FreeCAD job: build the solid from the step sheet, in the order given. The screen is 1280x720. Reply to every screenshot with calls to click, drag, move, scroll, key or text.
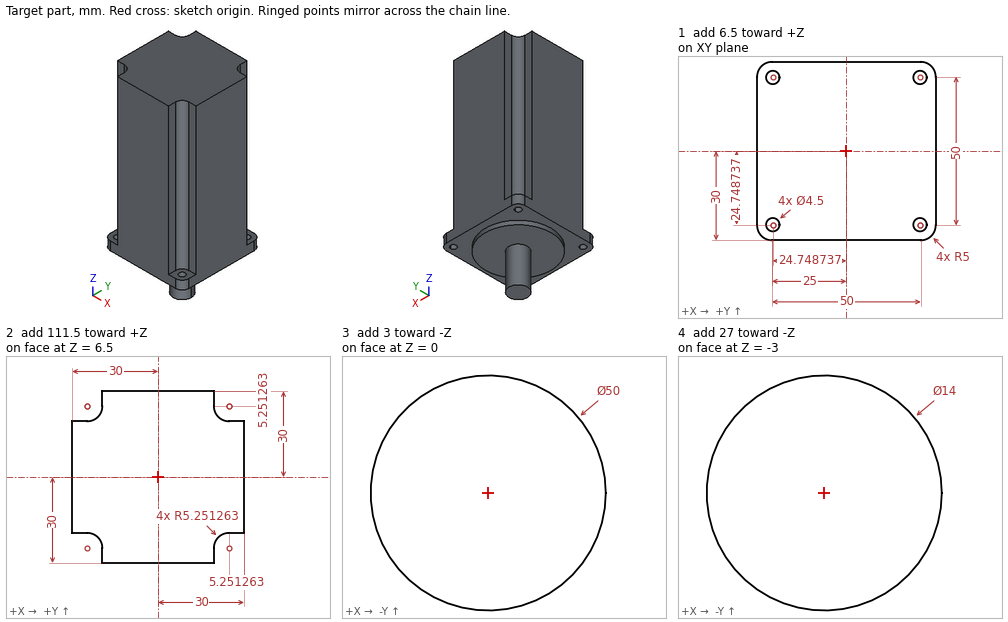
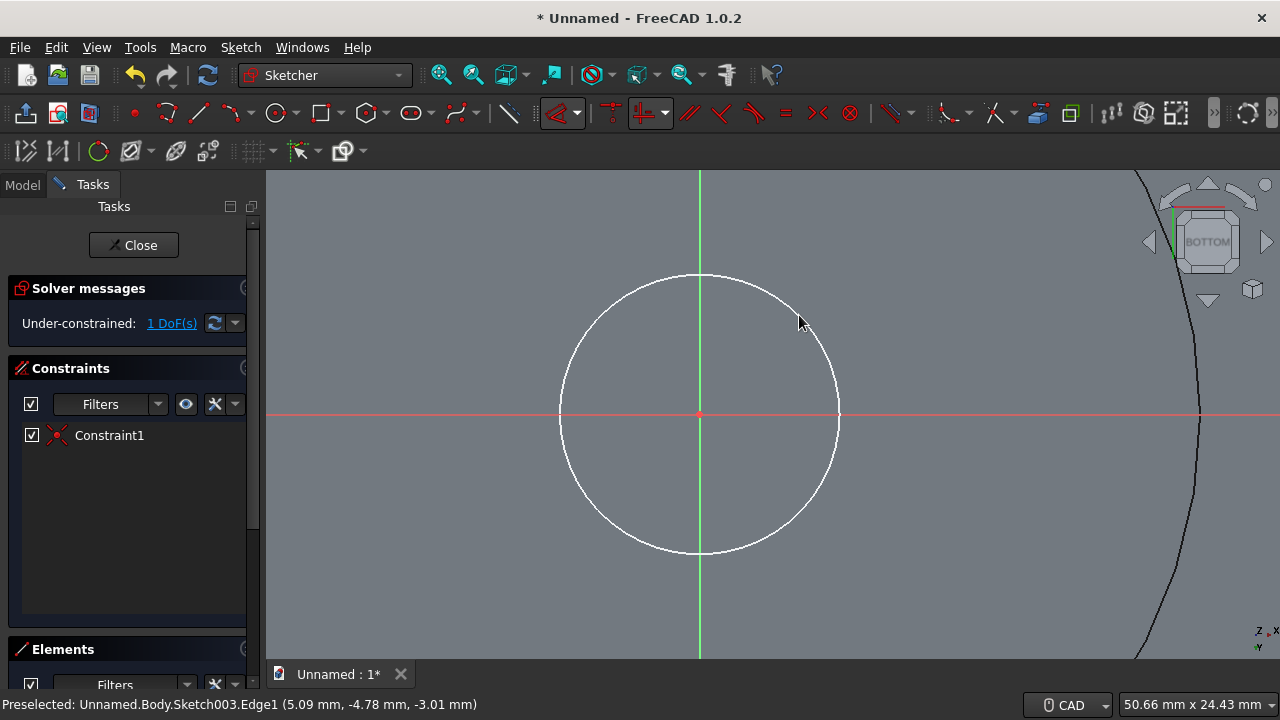
click(798, 315)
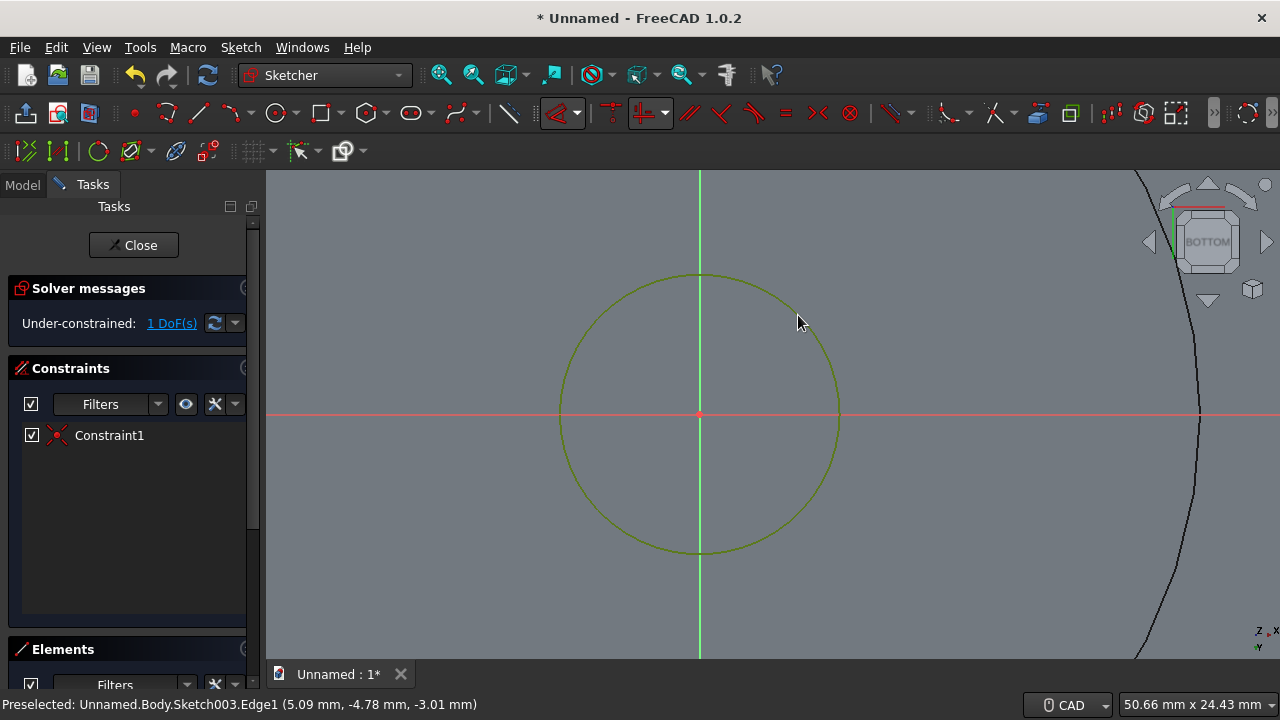
key(k)
key(o)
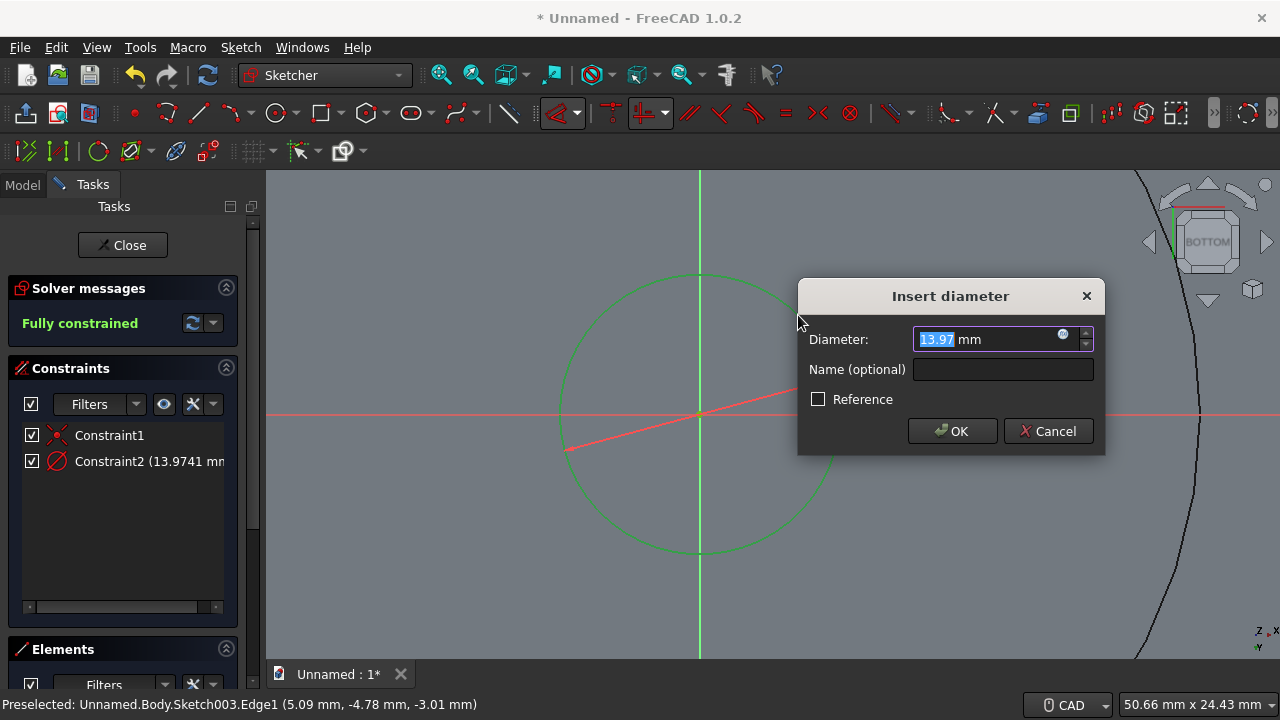
text(14)
key(Return)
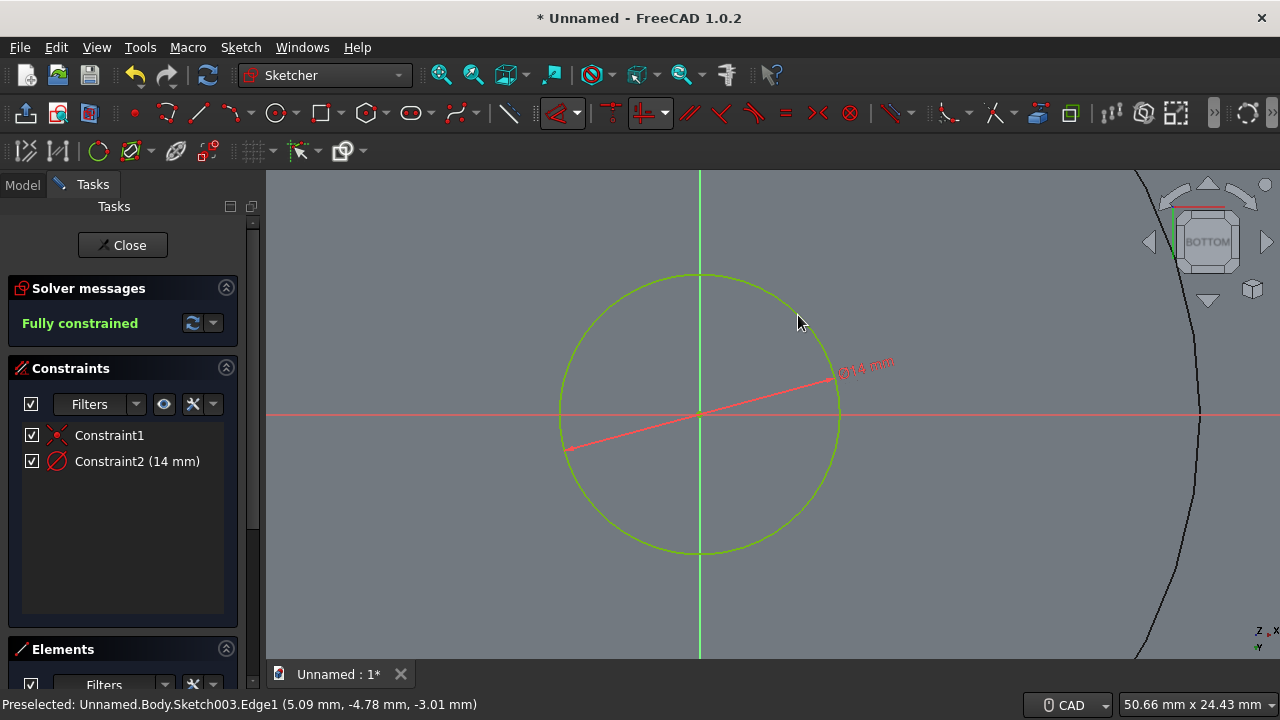
click(123, 245)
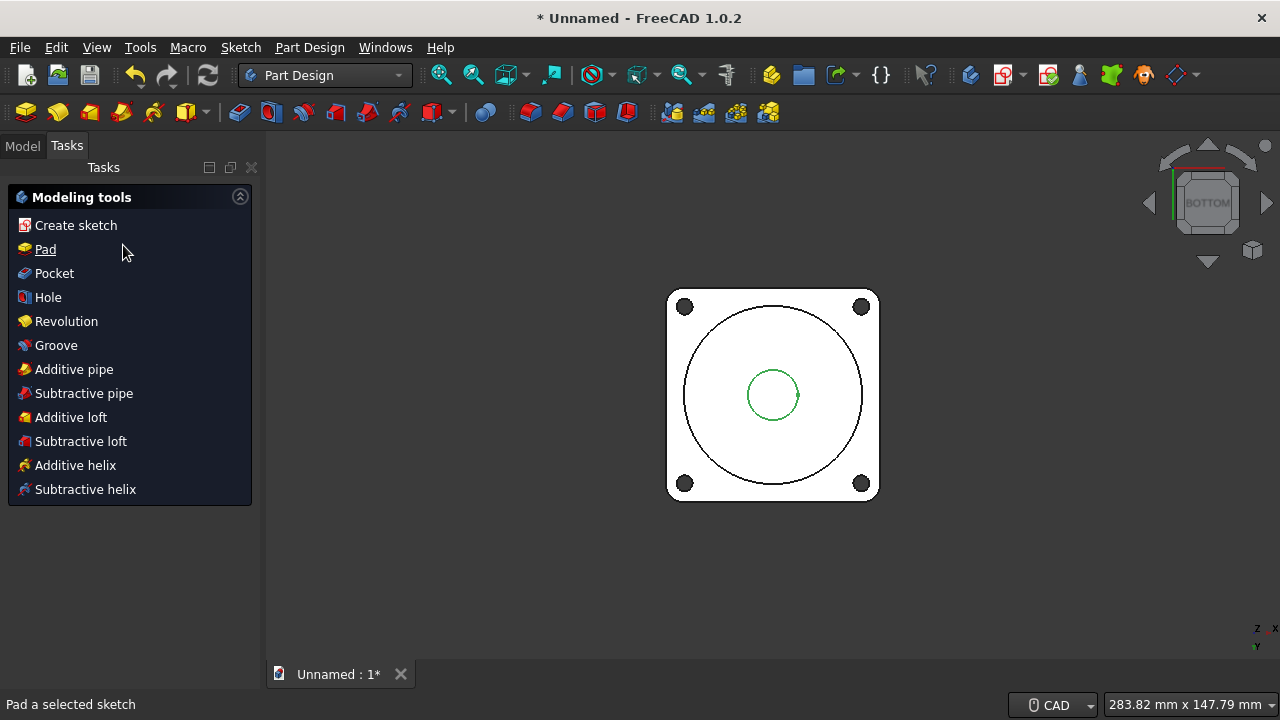
click(26, 112)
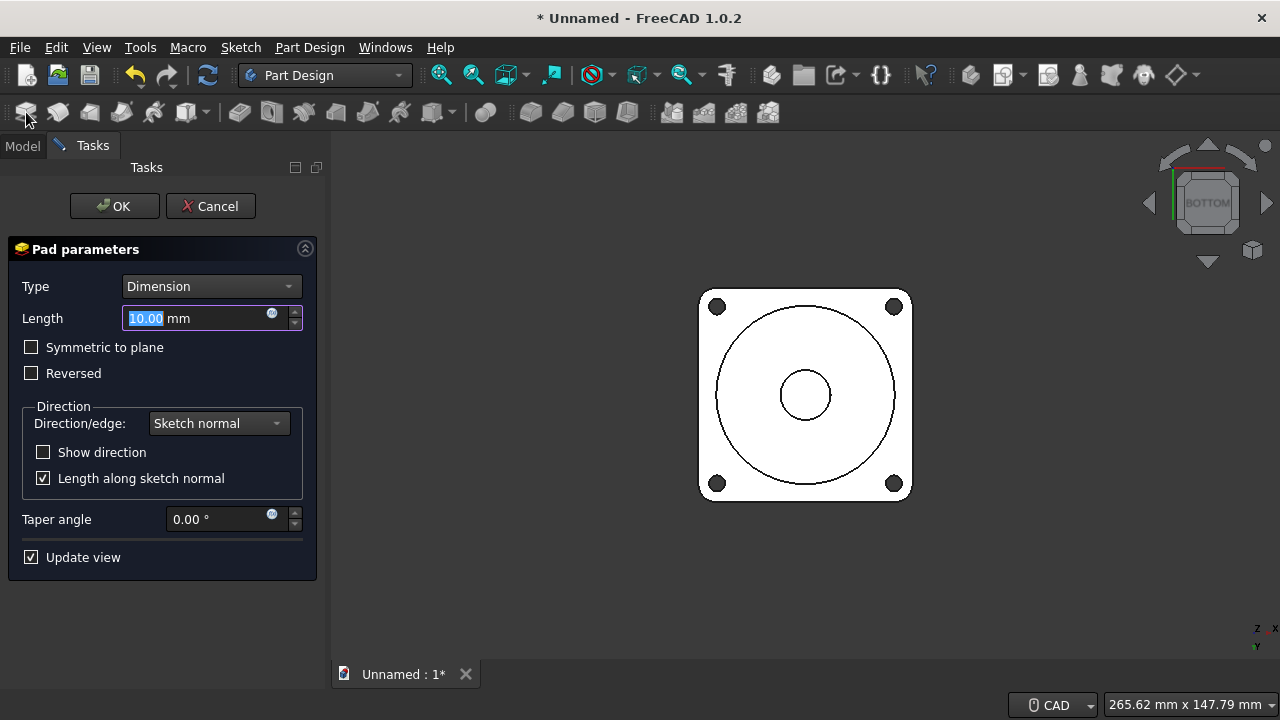
text(27)
key(Tab)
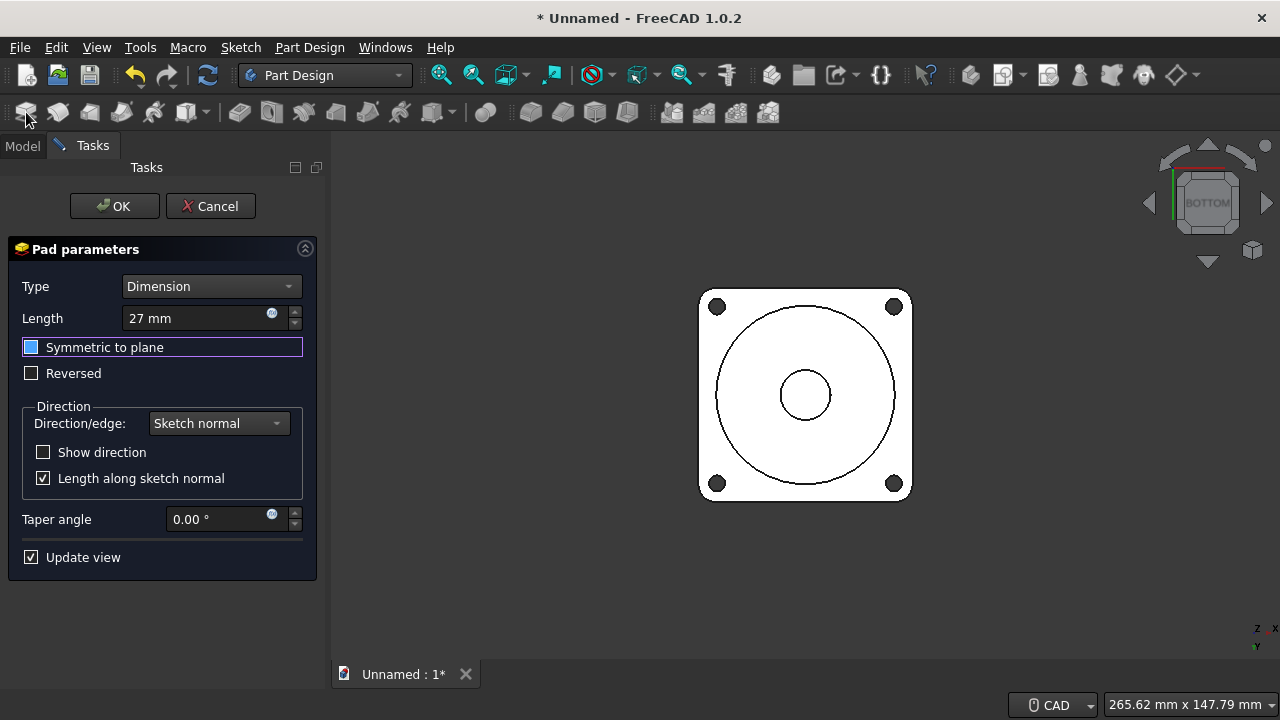
click(115, 206)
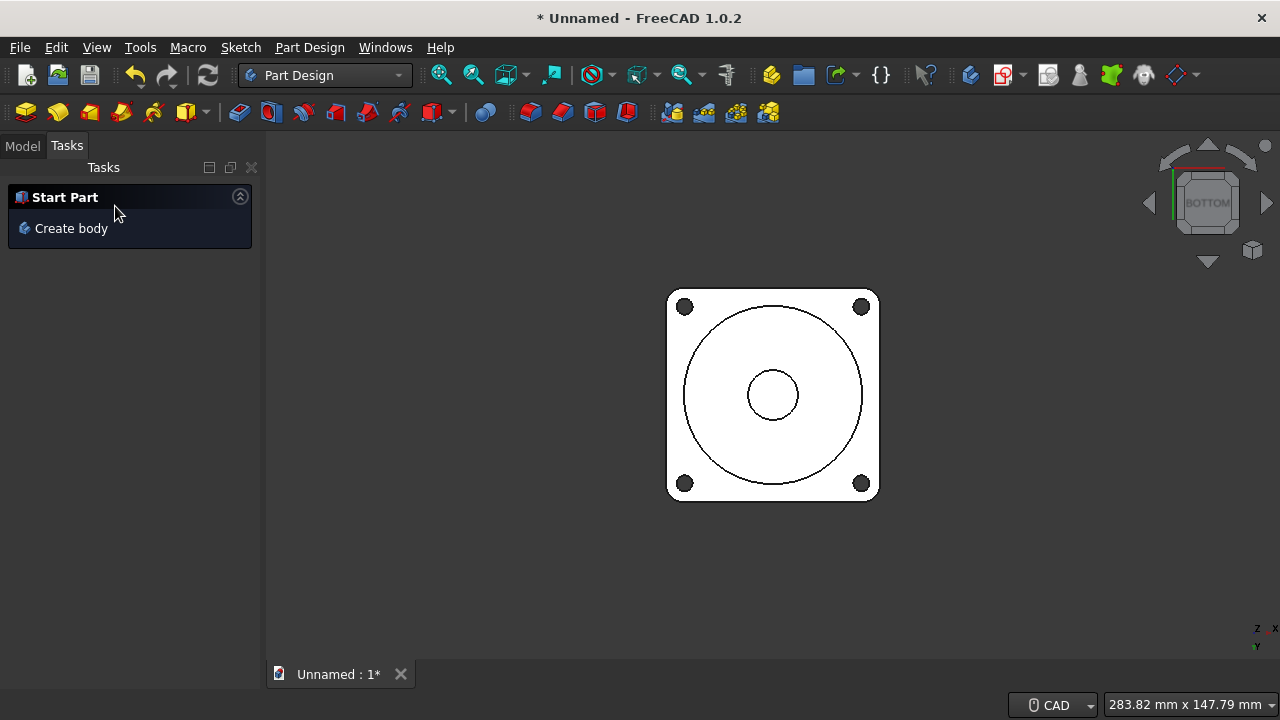
key(0)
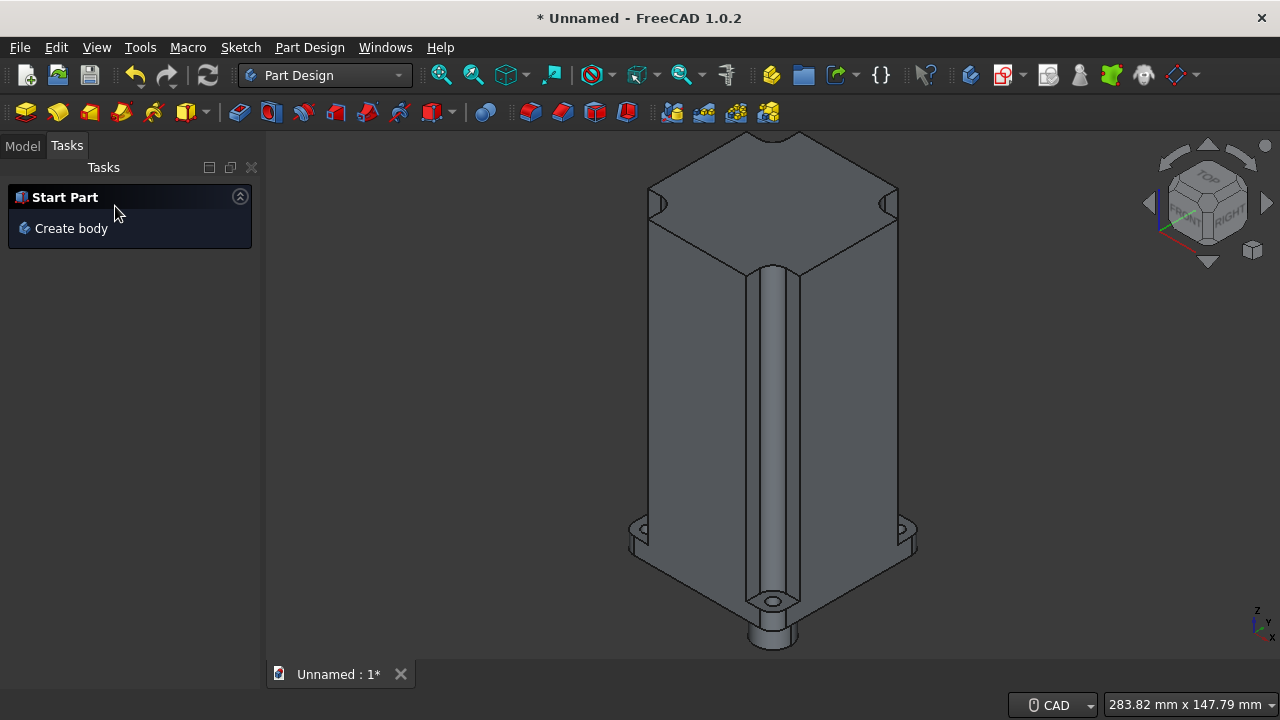
click(442, 76)